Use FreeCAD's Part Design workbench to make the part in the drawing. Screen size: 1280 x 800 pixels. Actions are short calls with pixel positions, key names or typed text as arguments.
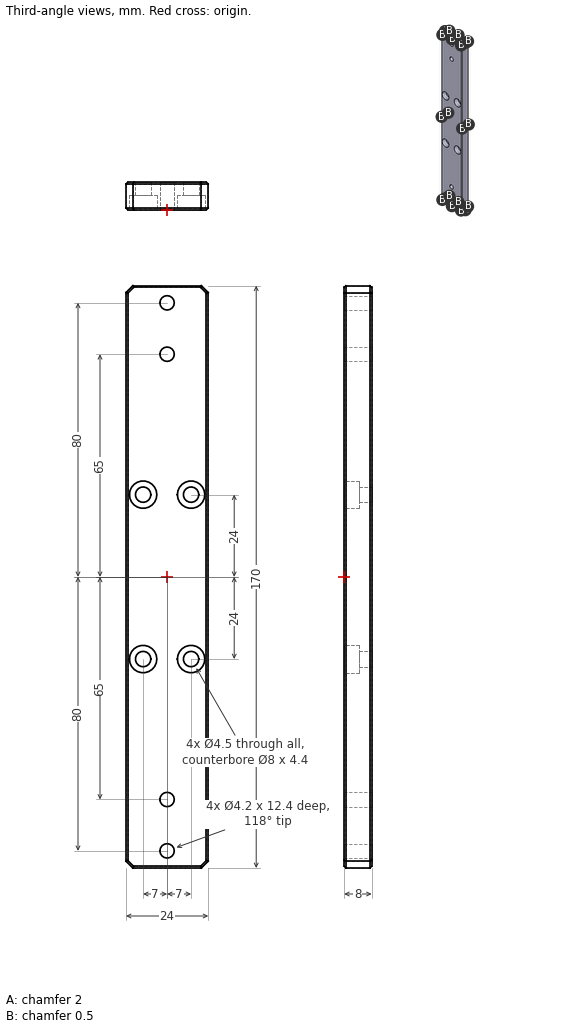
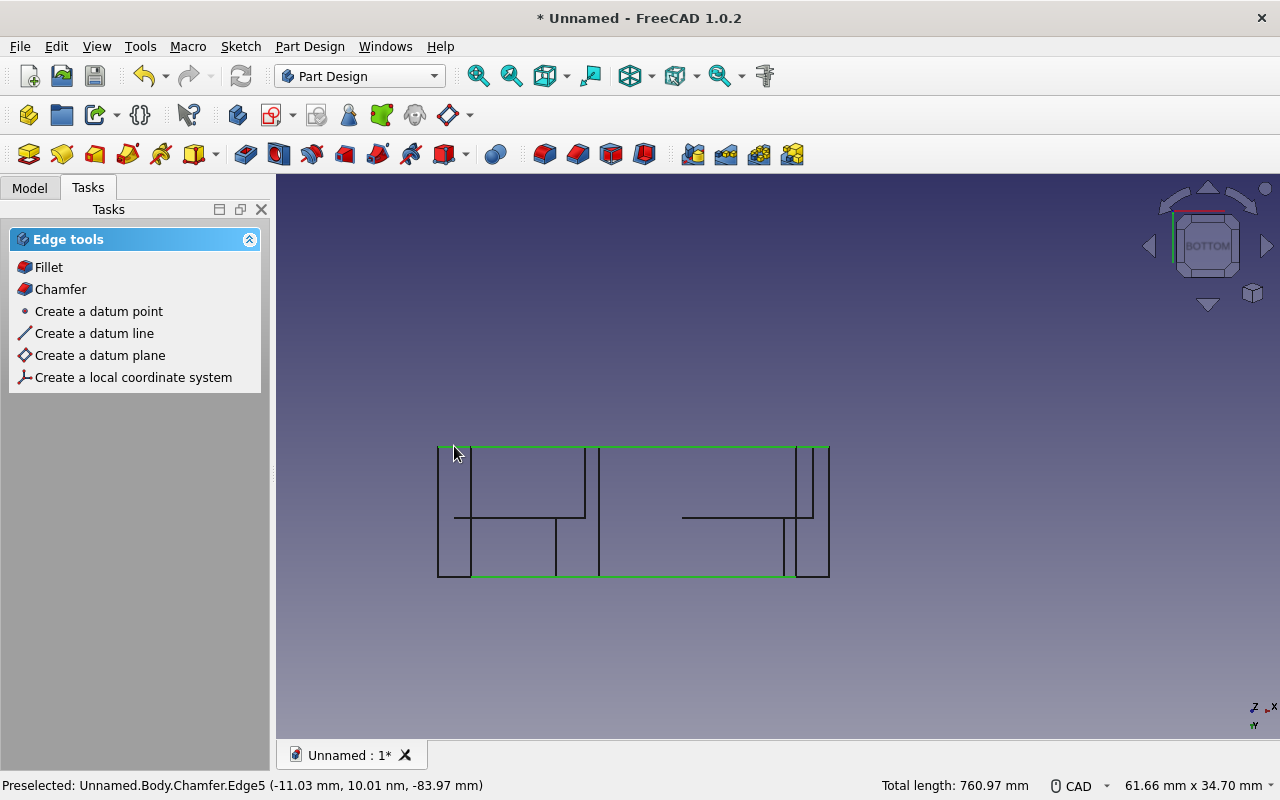
click(813, 576, ctrl)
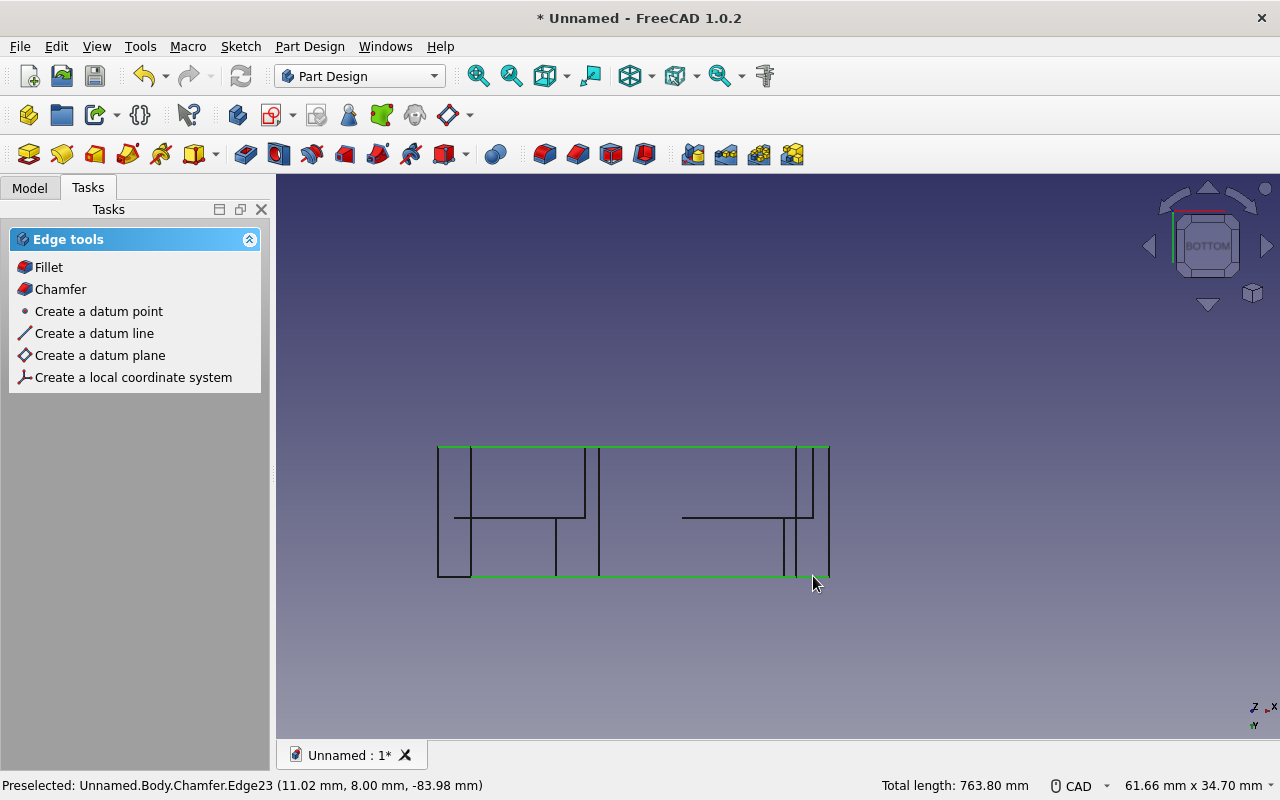
click(454, 576, ctrl)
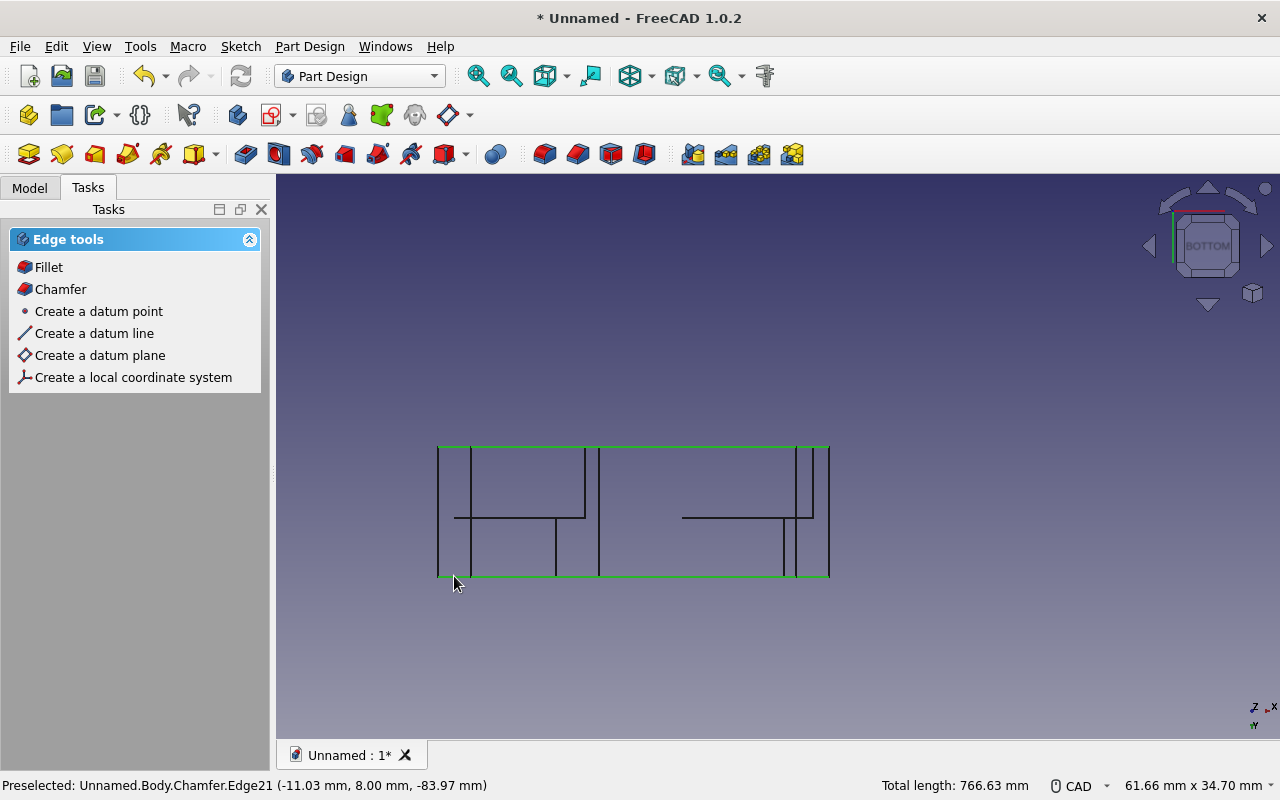
key(v)
key(1)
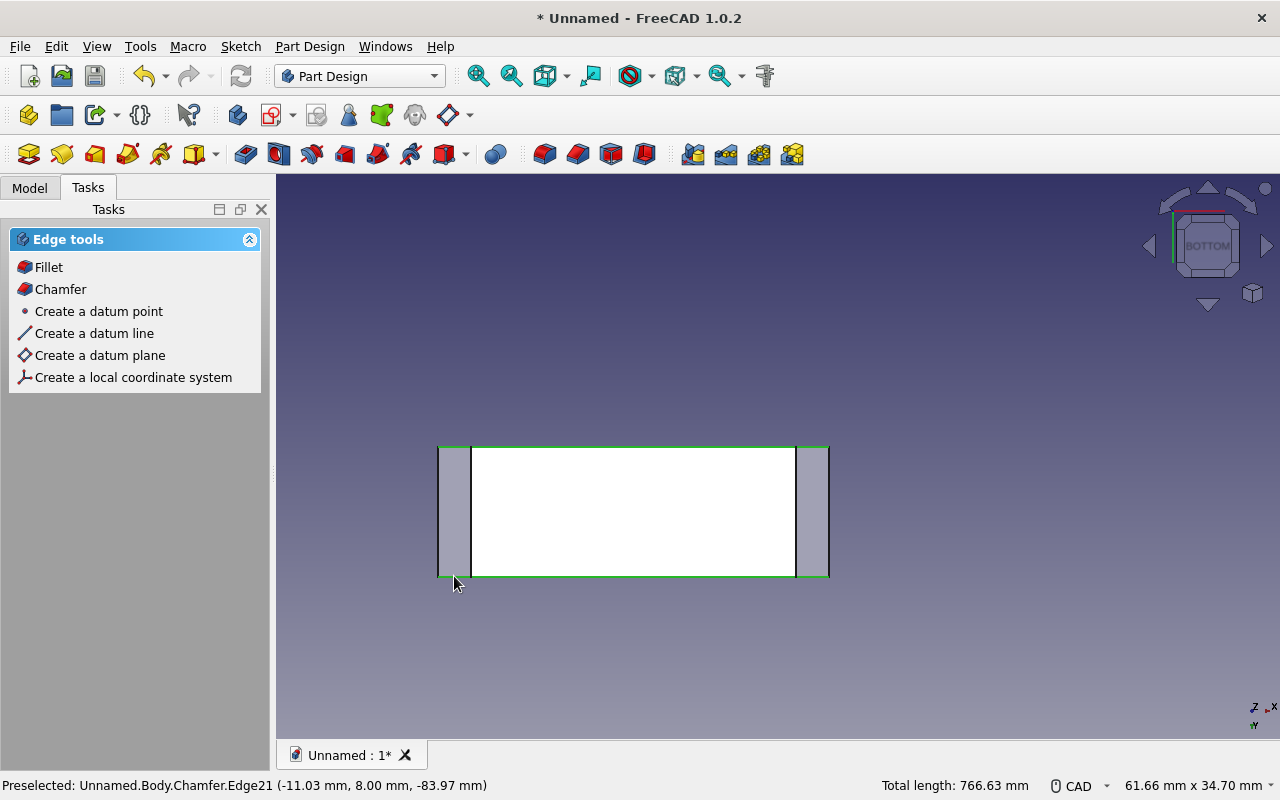
click(578, 154)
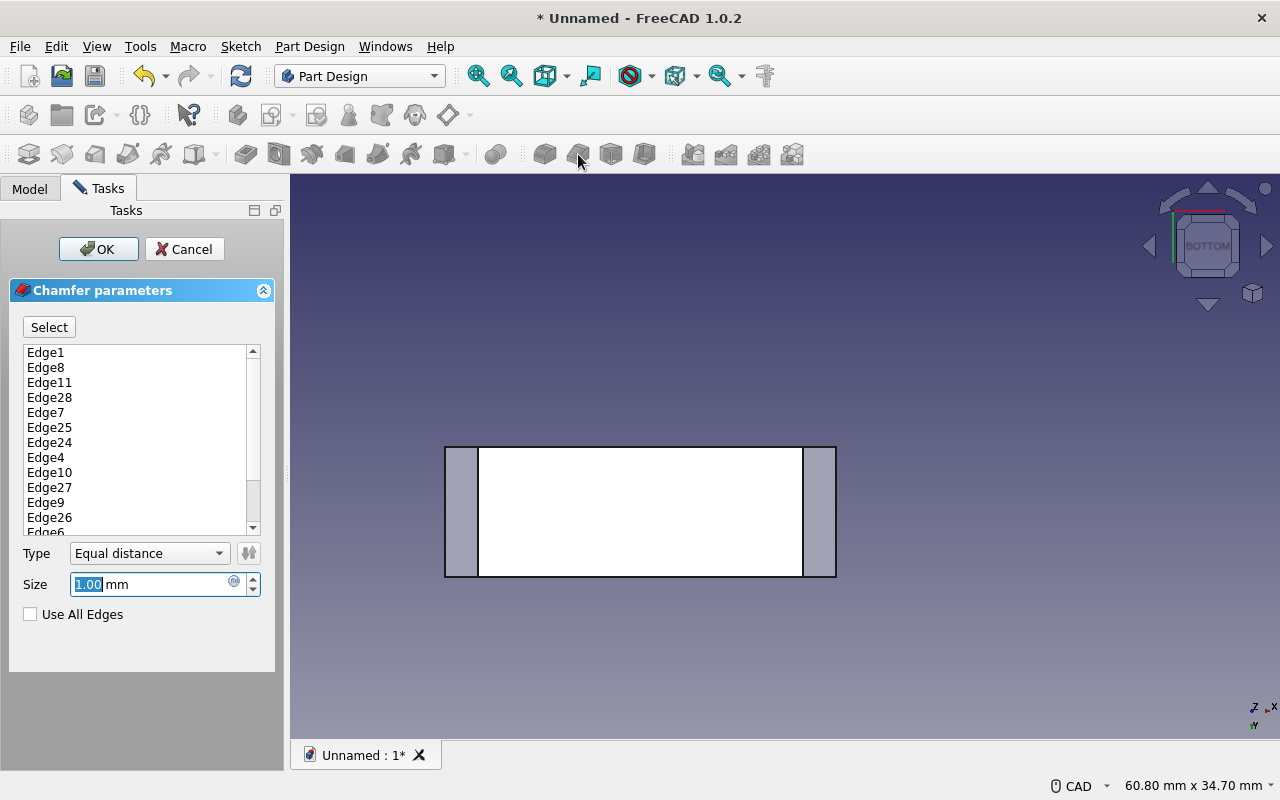
text(0.5)
key(Tab)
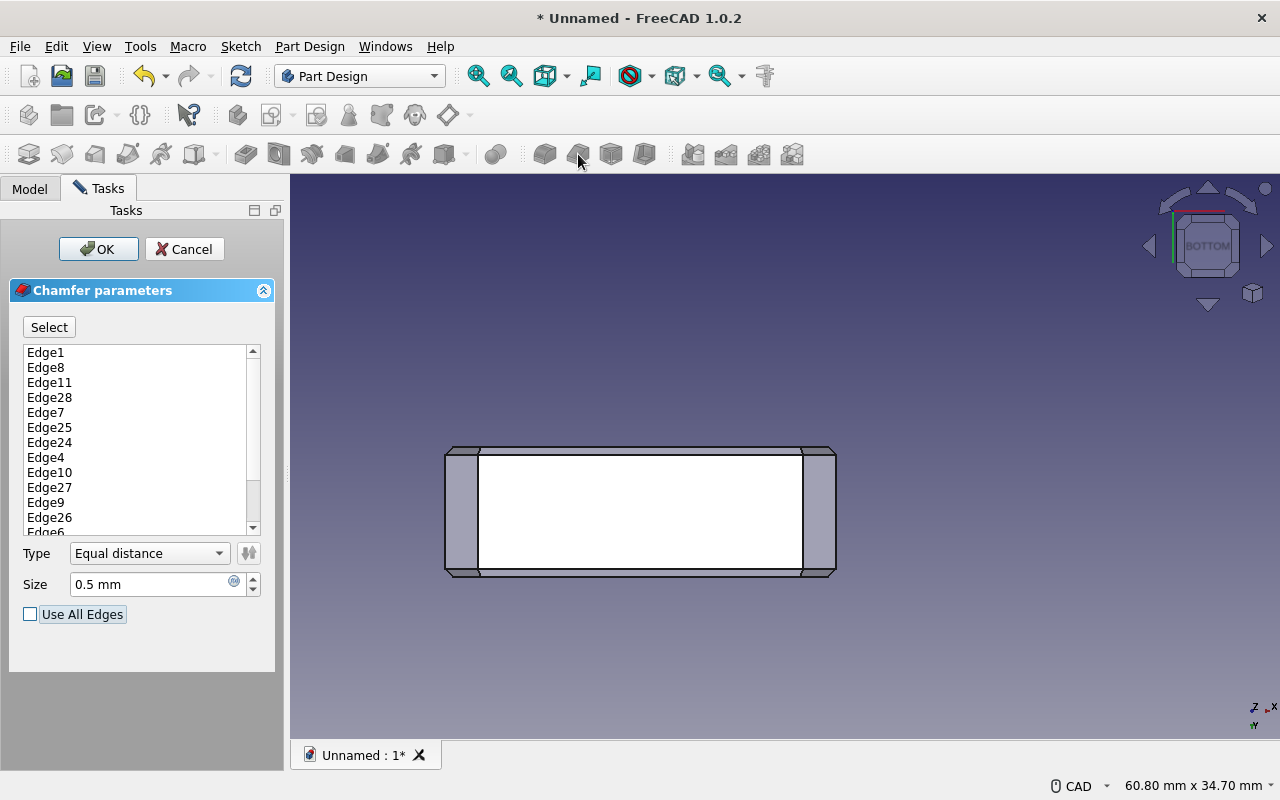
click(99, 249)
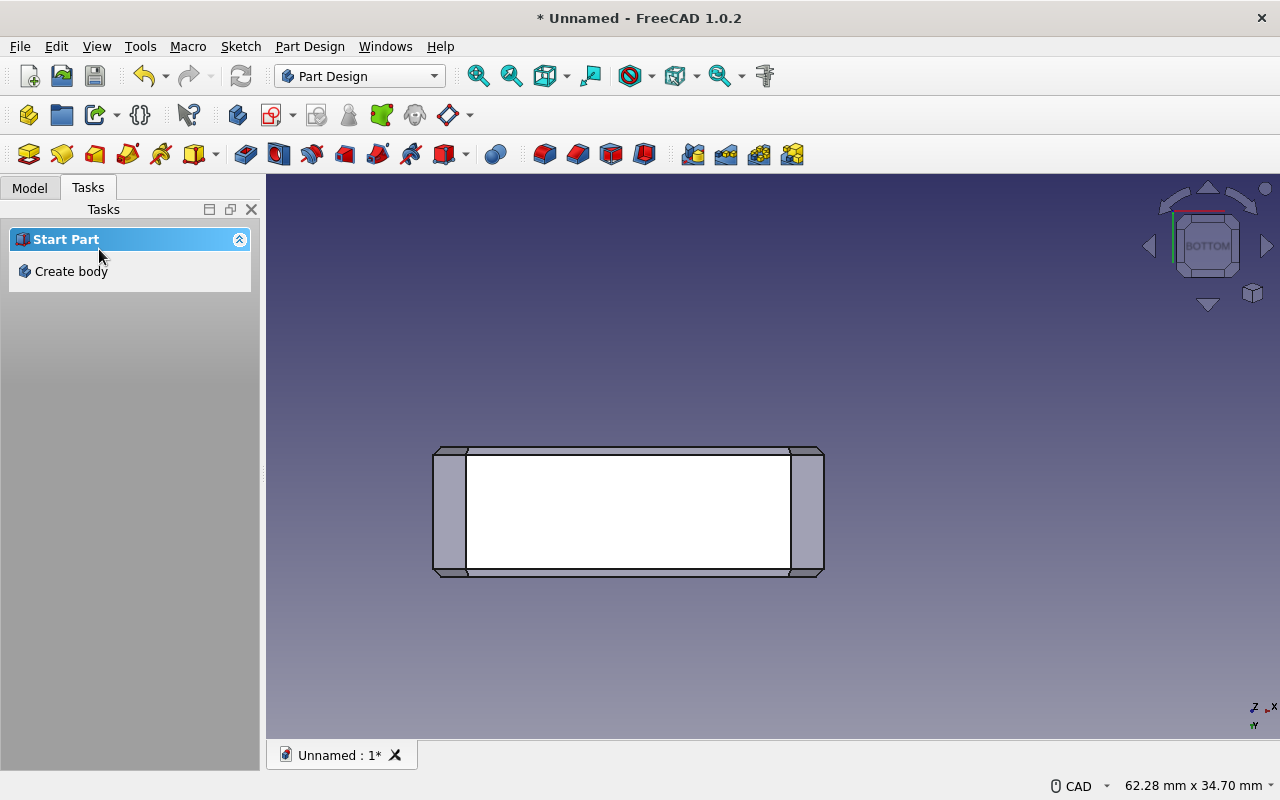
key(0)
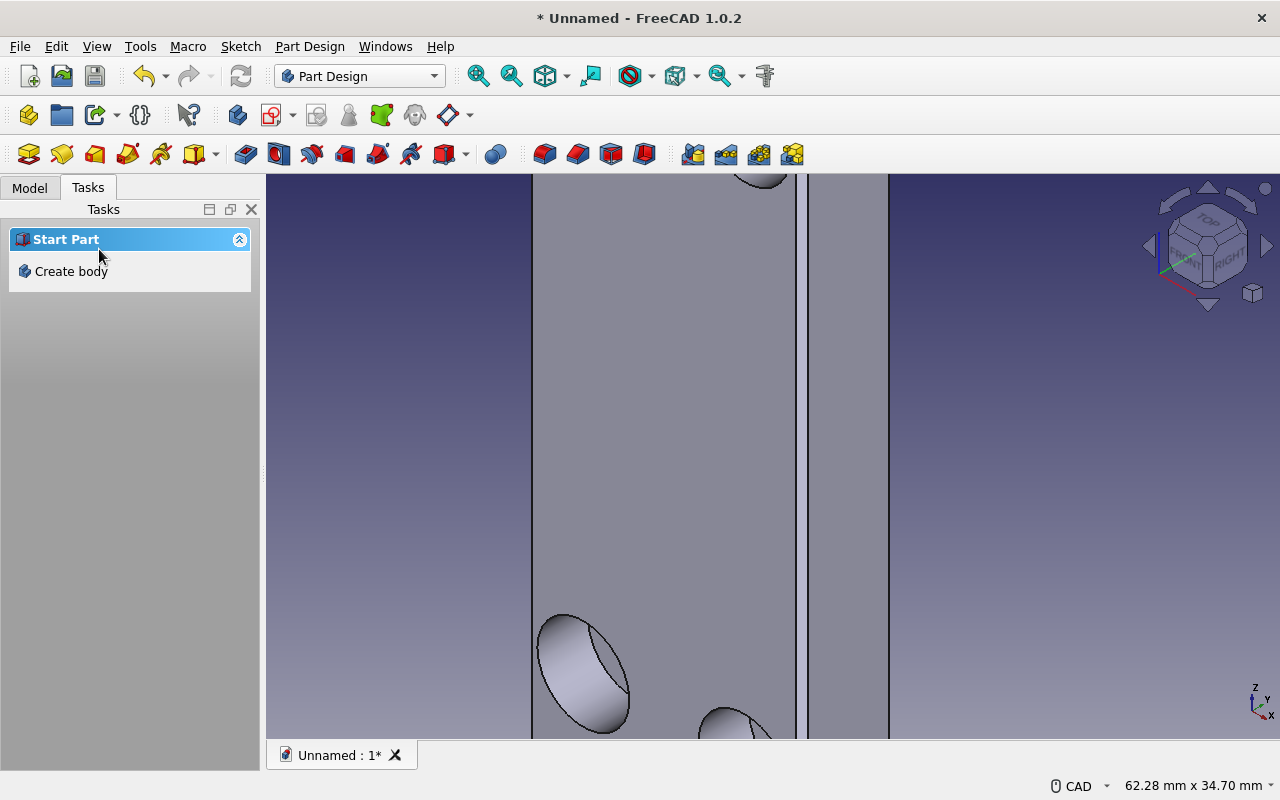
click(479, 76)